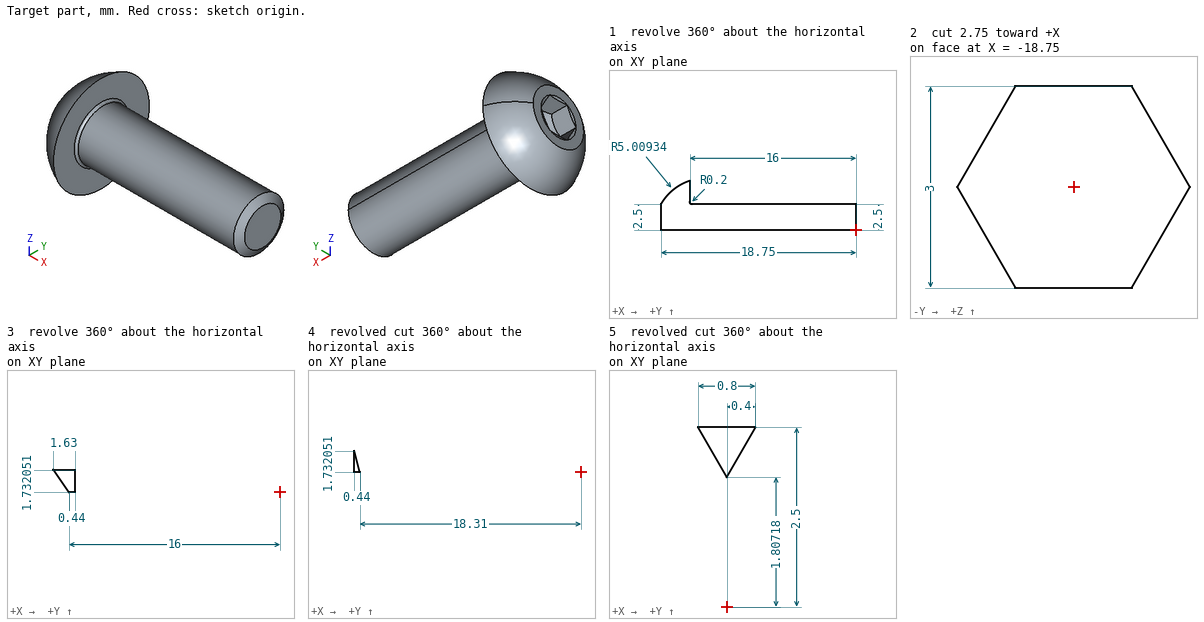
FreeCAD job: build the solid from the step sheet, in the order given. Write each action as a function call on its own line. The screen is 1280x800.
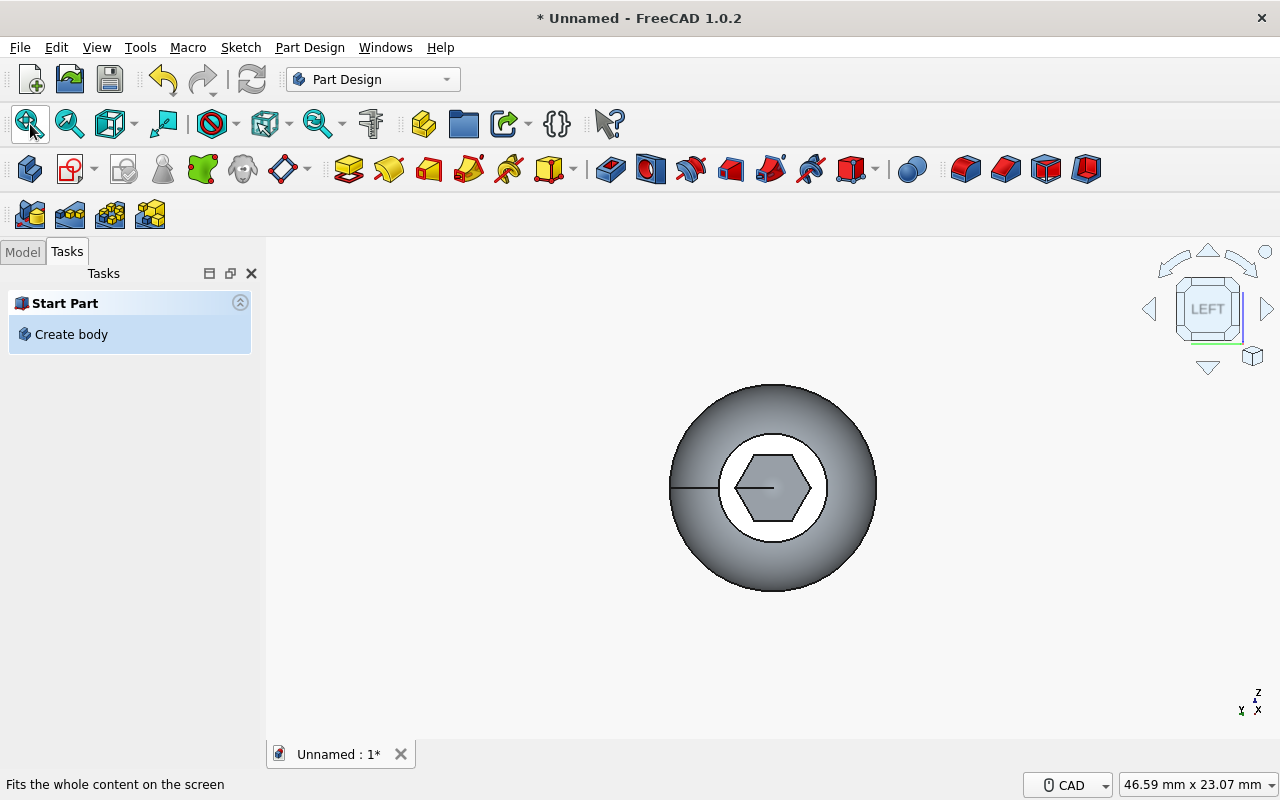
click(70, 170)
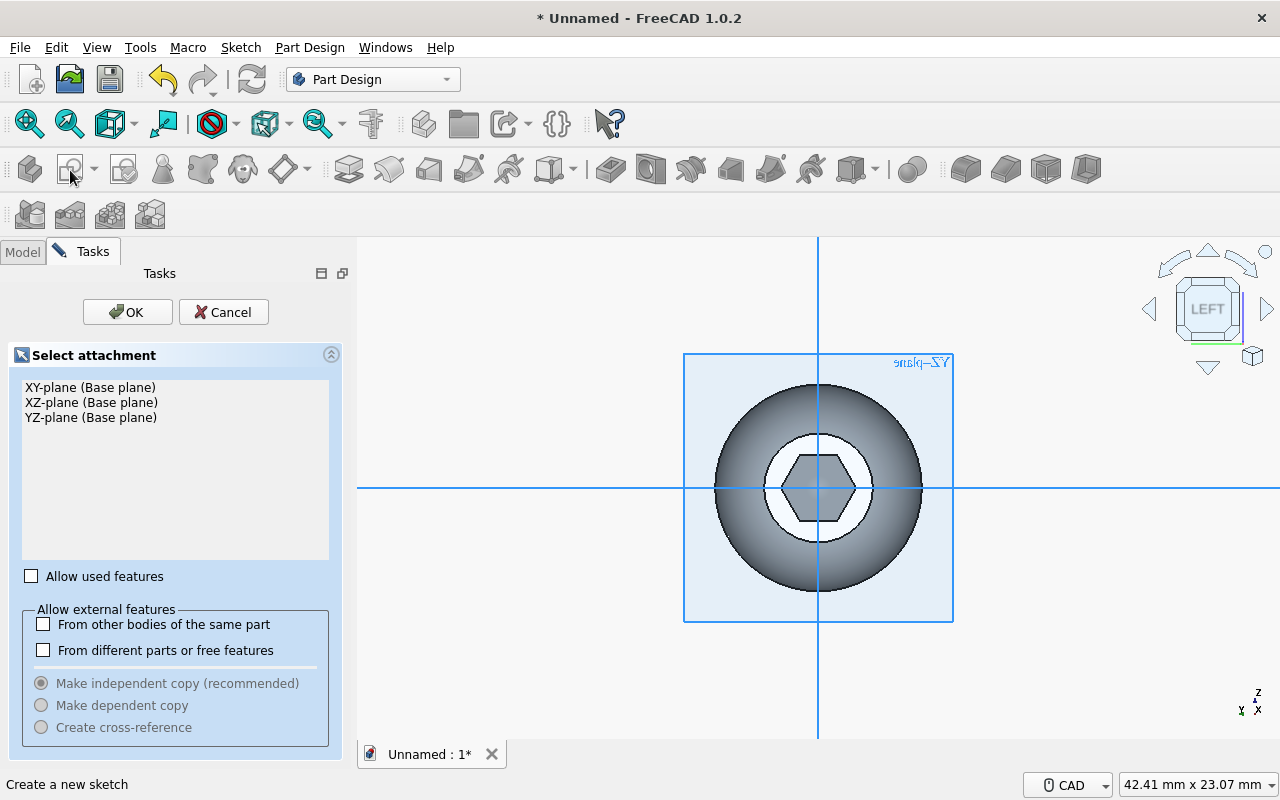
click(82, 388)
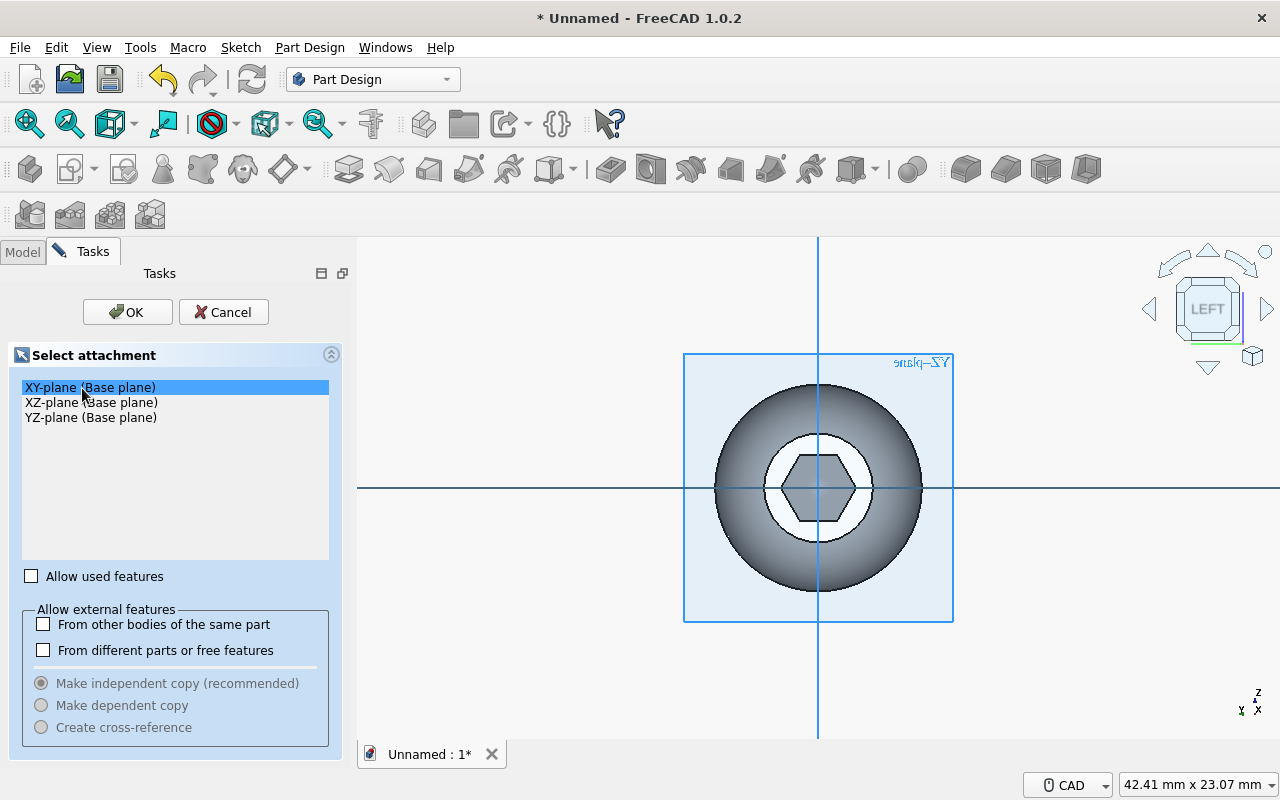
click(128, 312)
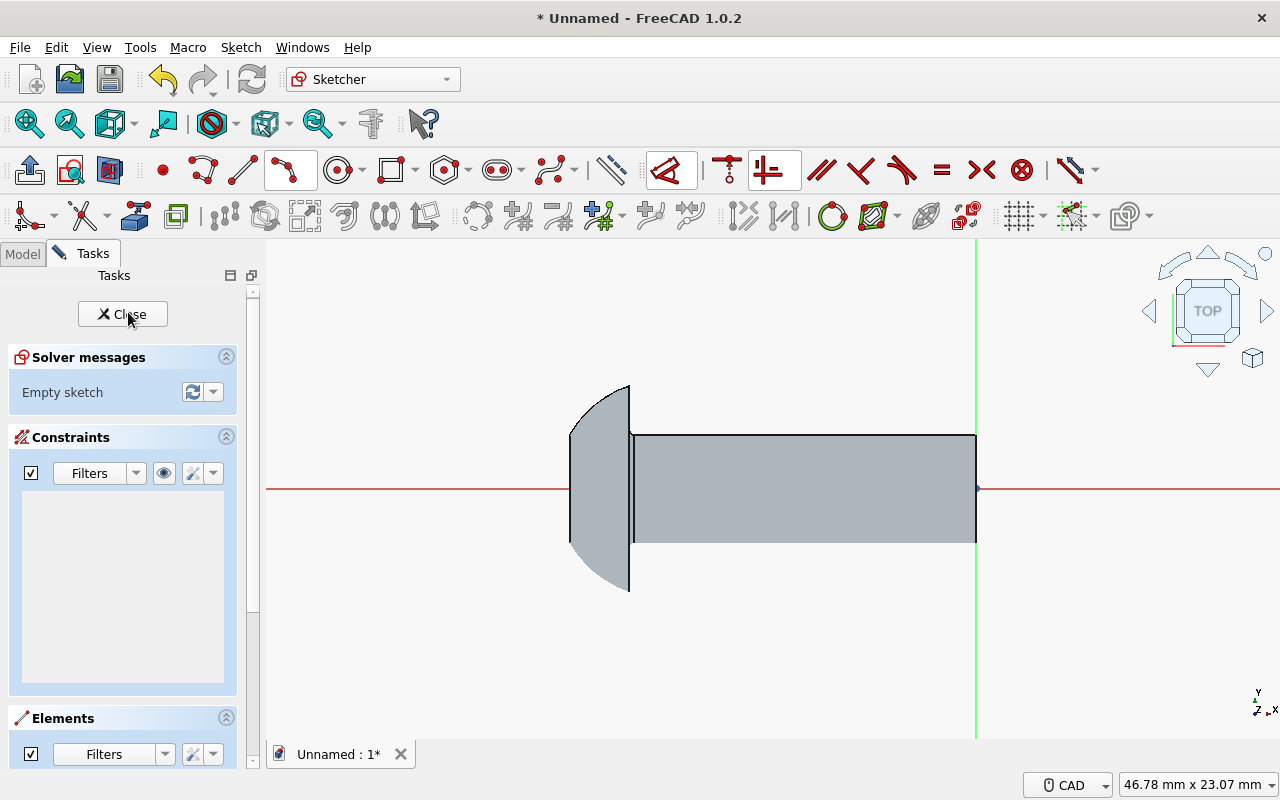
click(110, 170)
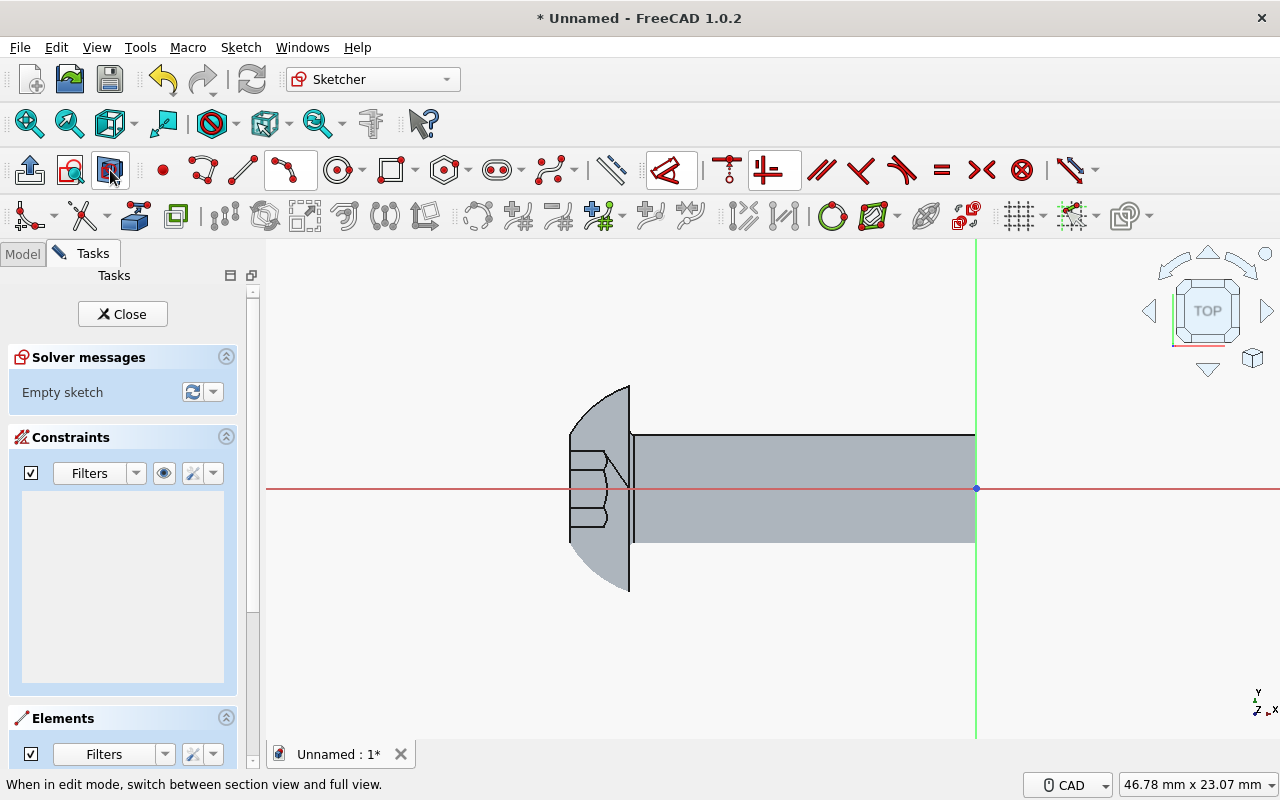
scroll(558, 468, up, 11)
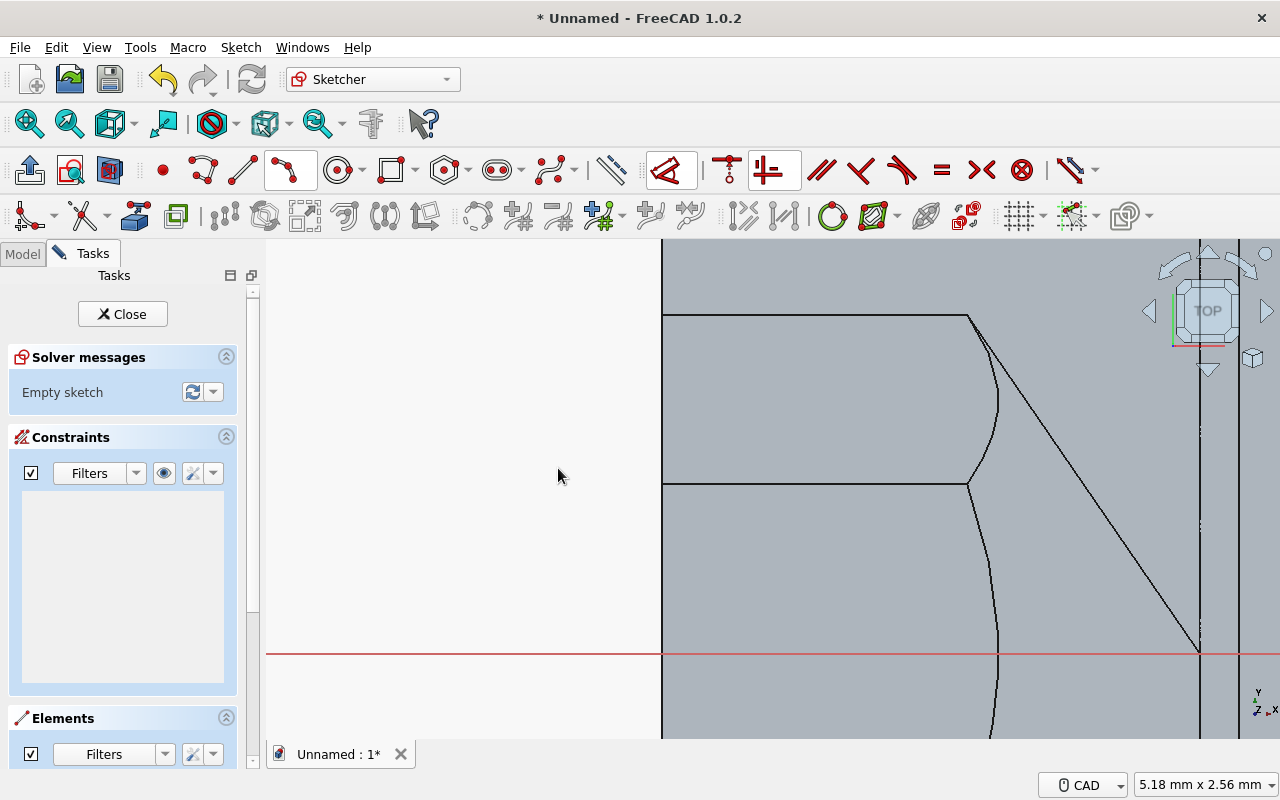
click(204, 170)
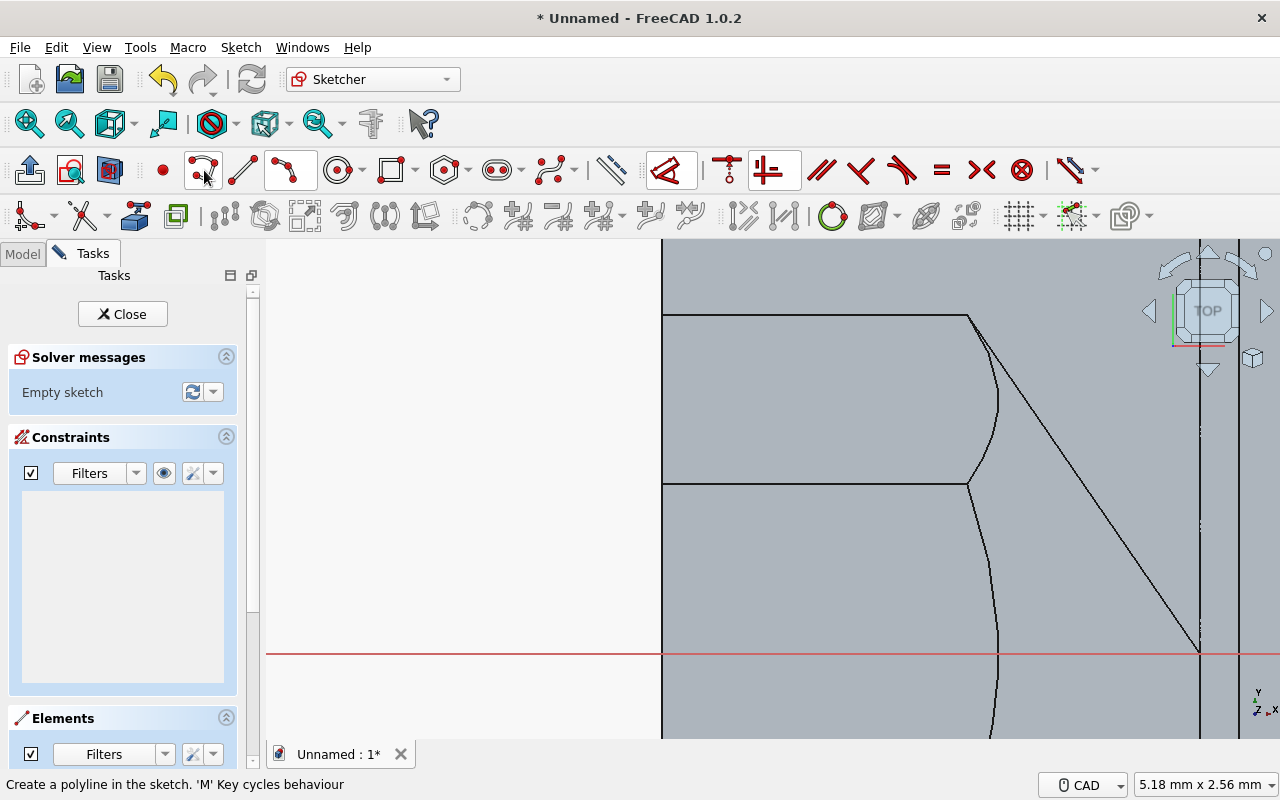
click(748, 654)
click(662, 315)
click(662, 645)
click(748, 654)
key(Escape)
key(Escape)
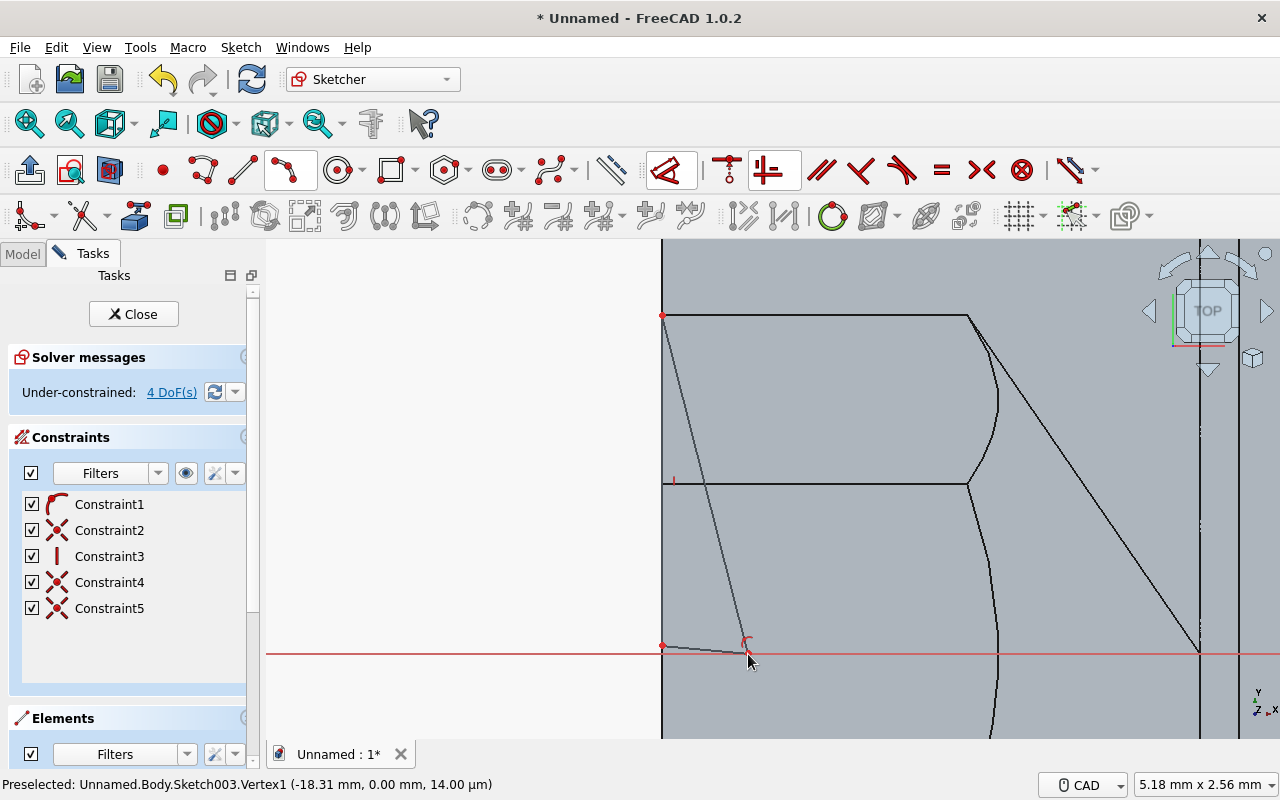
click(722, 651)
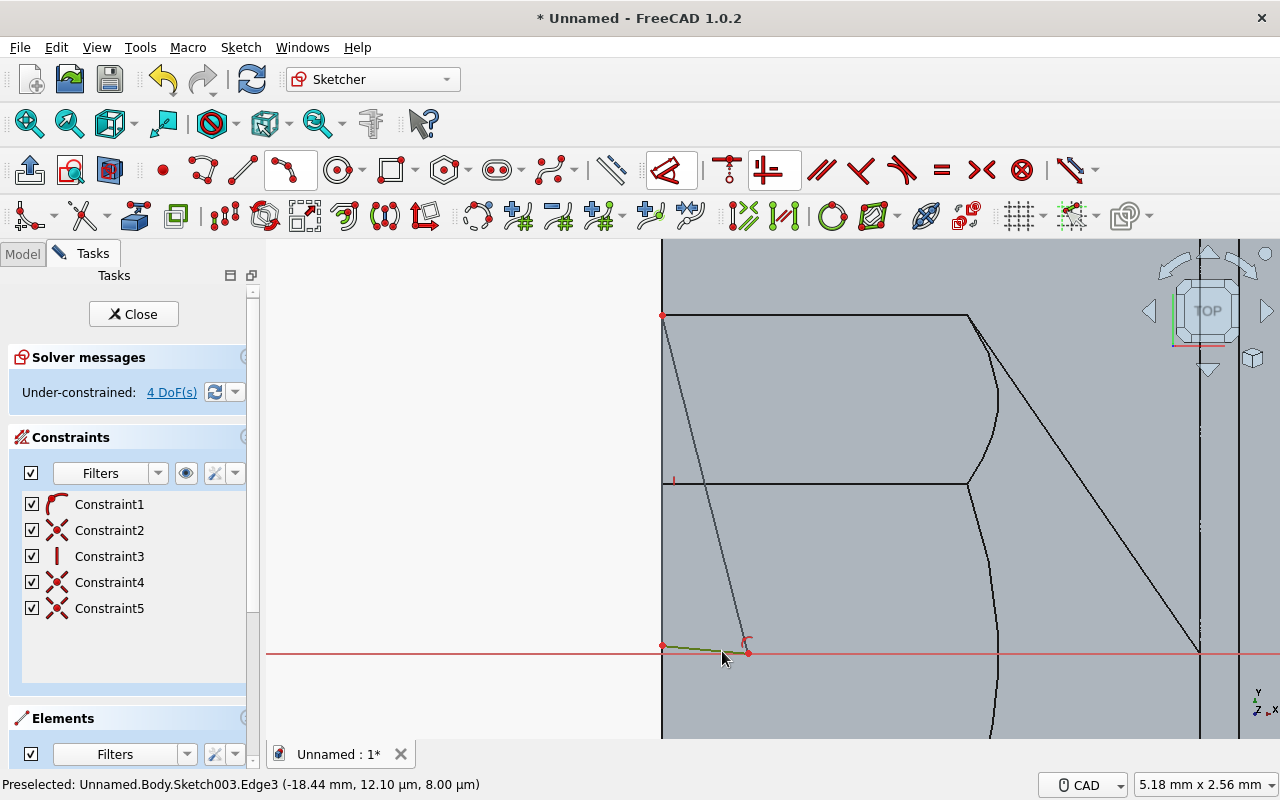
key(h)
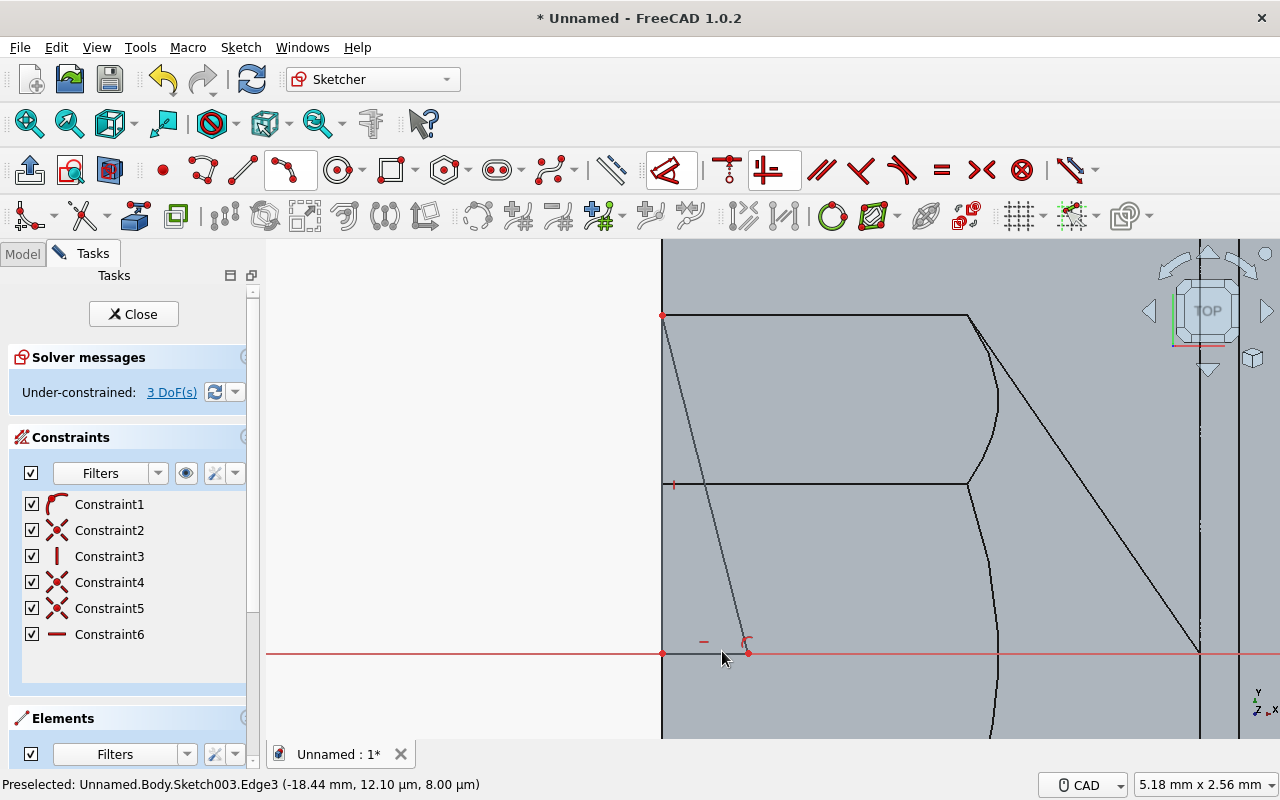
click(688, 654)